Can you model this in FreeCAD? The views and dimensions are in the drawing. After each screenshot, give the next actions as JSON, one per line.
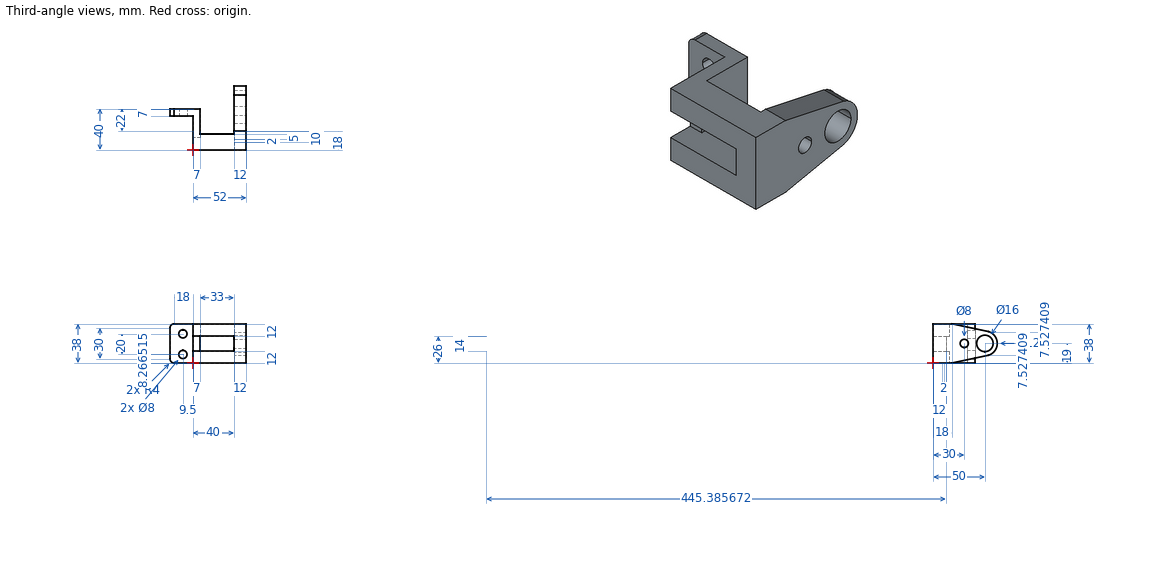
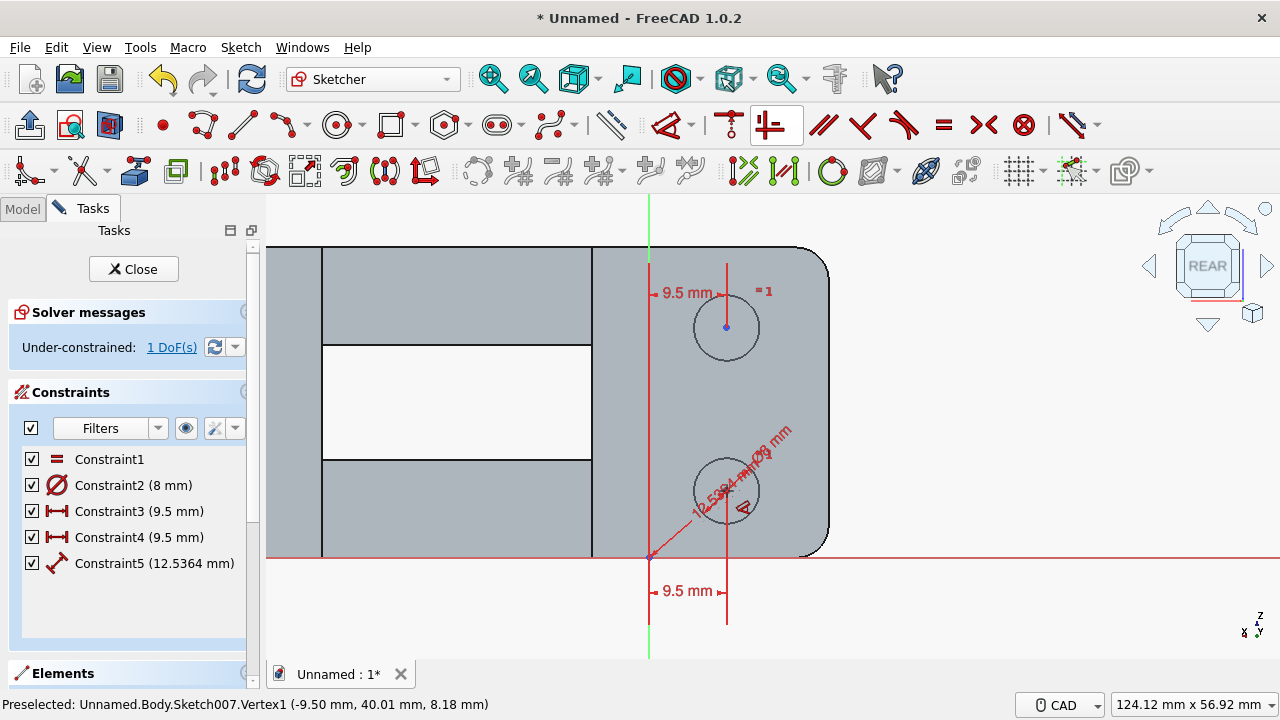
{"action": "left_click", "coordinate": [727, 328]}
{"action": "left_click", "coordinate": [761, 410]}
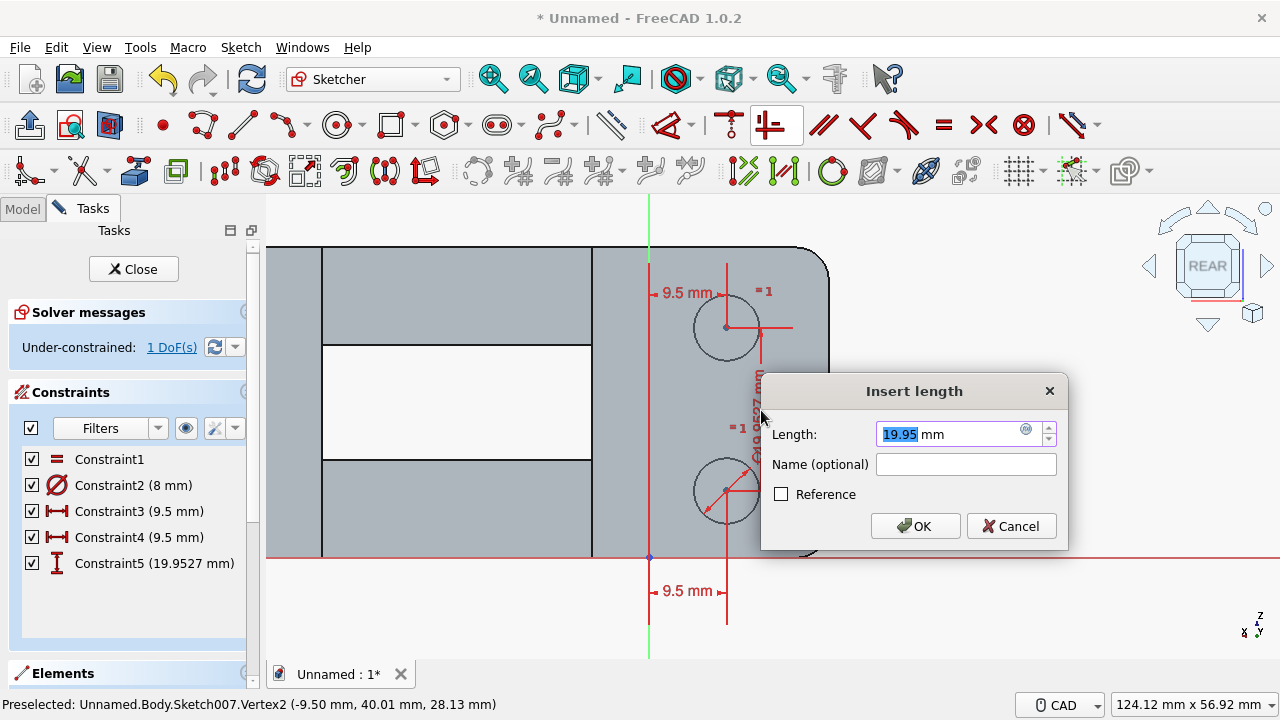
{"action": "type", "text": "20"}
{"action": "key", "text": "Return"}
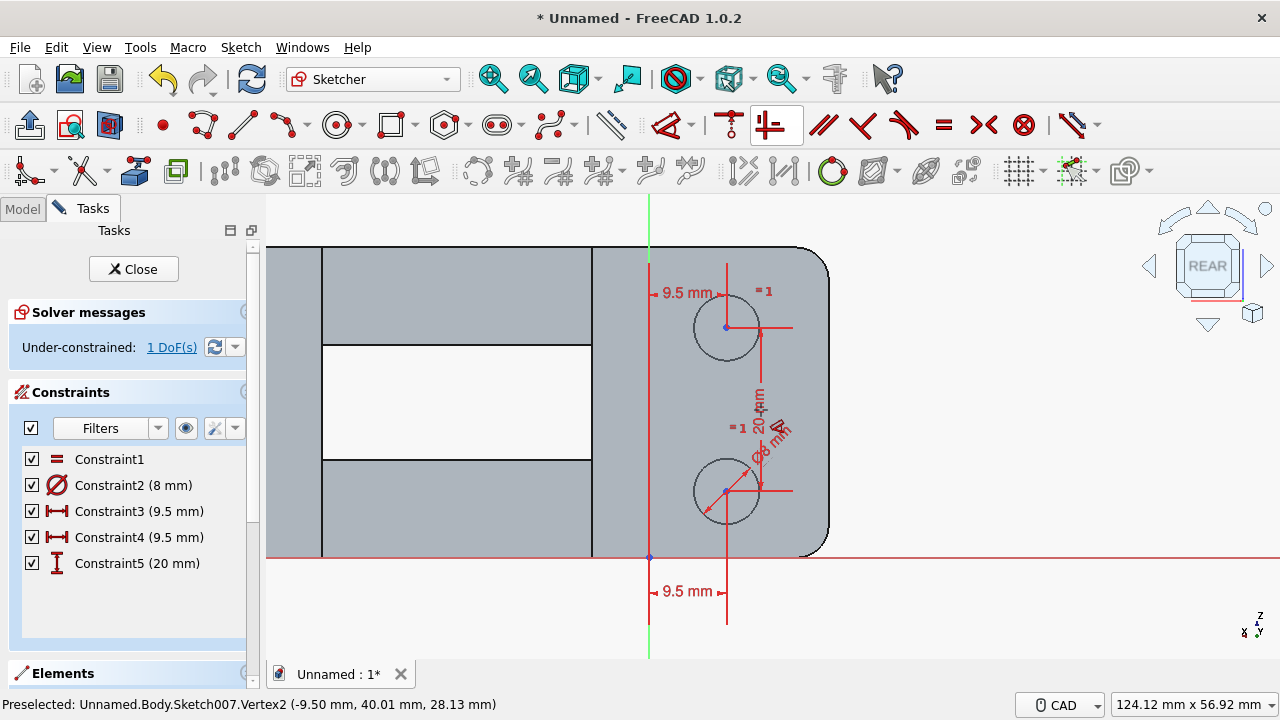
{"action": "left_click", "coordinate": [727, 491]}
{"action": "left_click", "coordinate": [615, 525]}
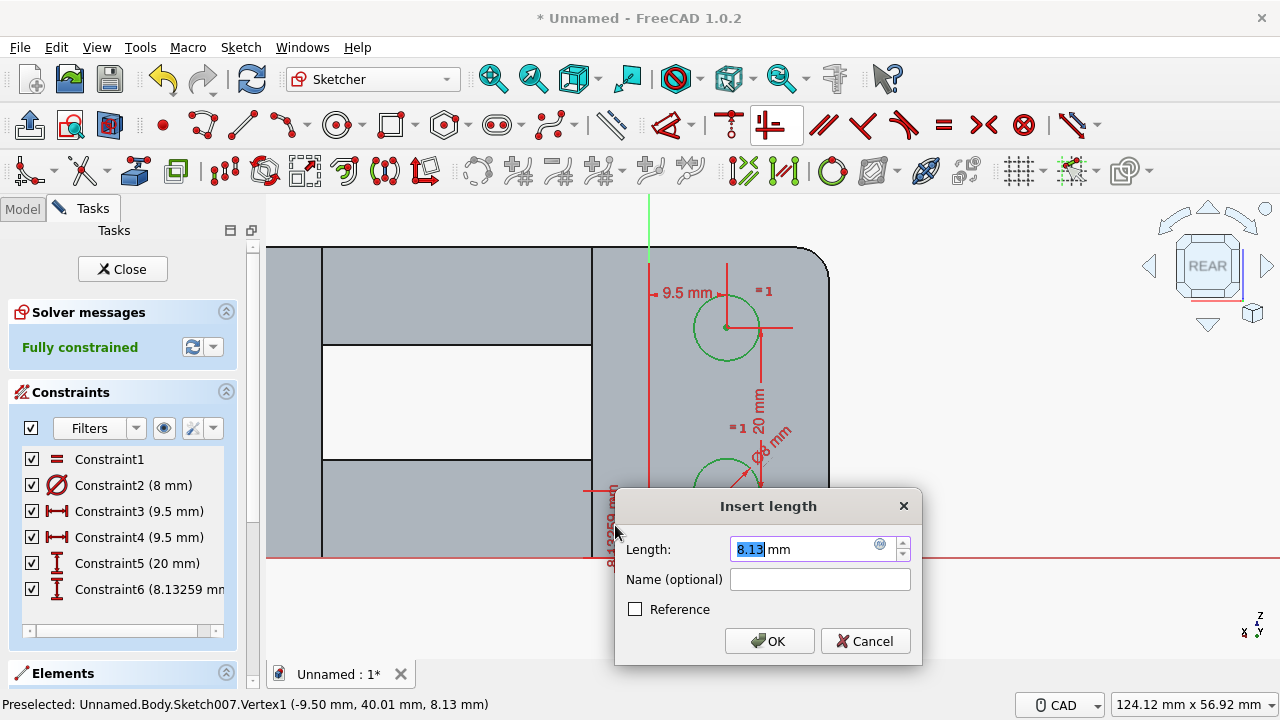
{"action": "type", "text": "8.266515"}
{"action": "key", "text": "Return"}
{"action": "key", "text": "Escape"}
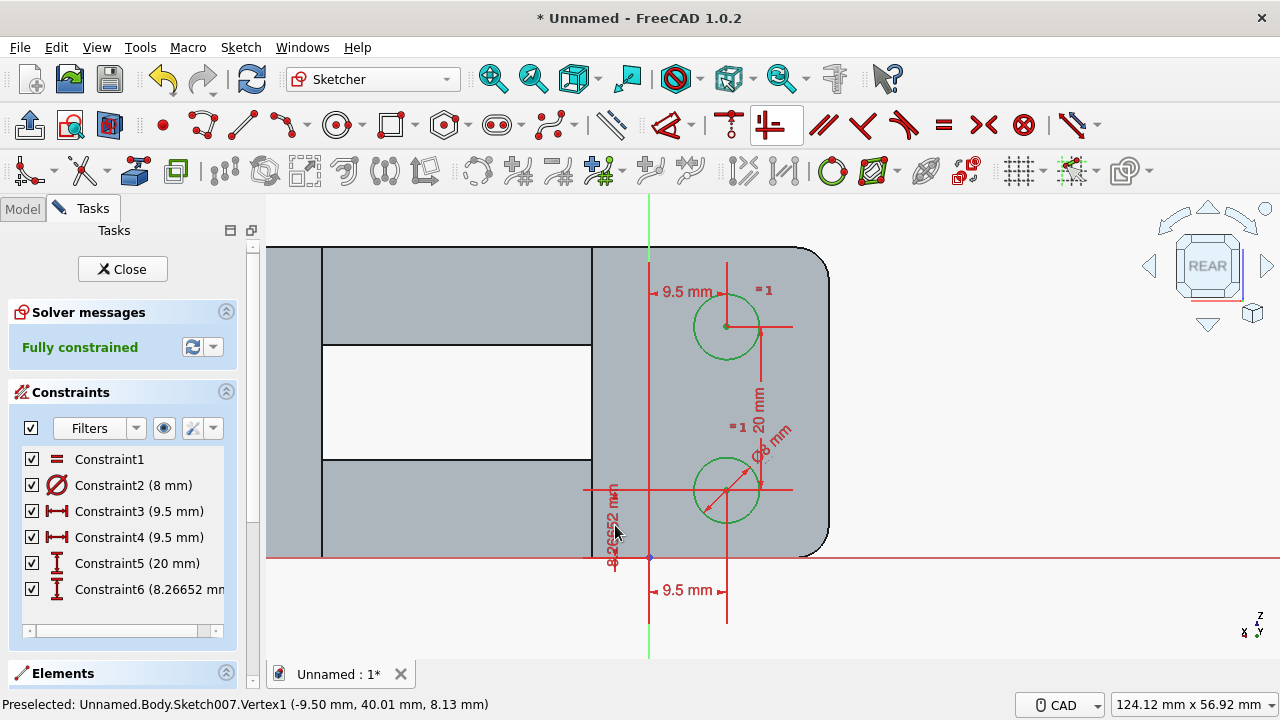
{"action": "left_click", "coordinate": [123, 269]}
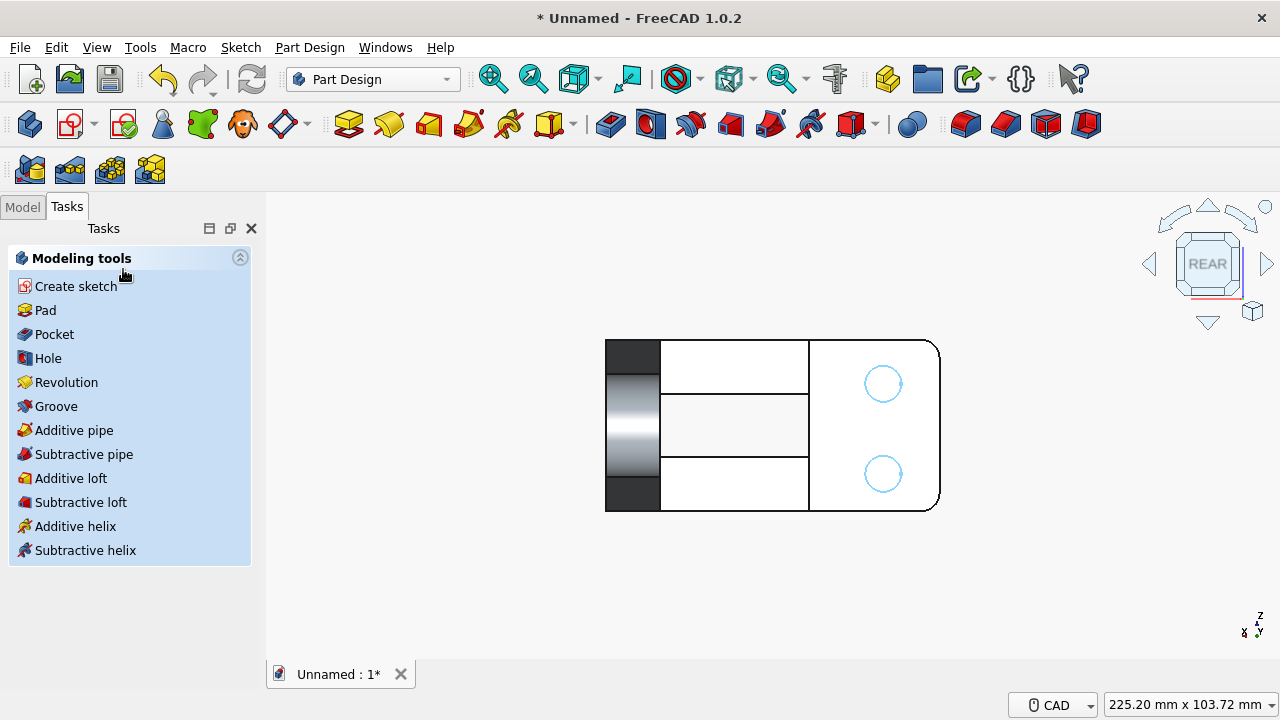
{"action": "left_click", "coordinate": [612, 124]}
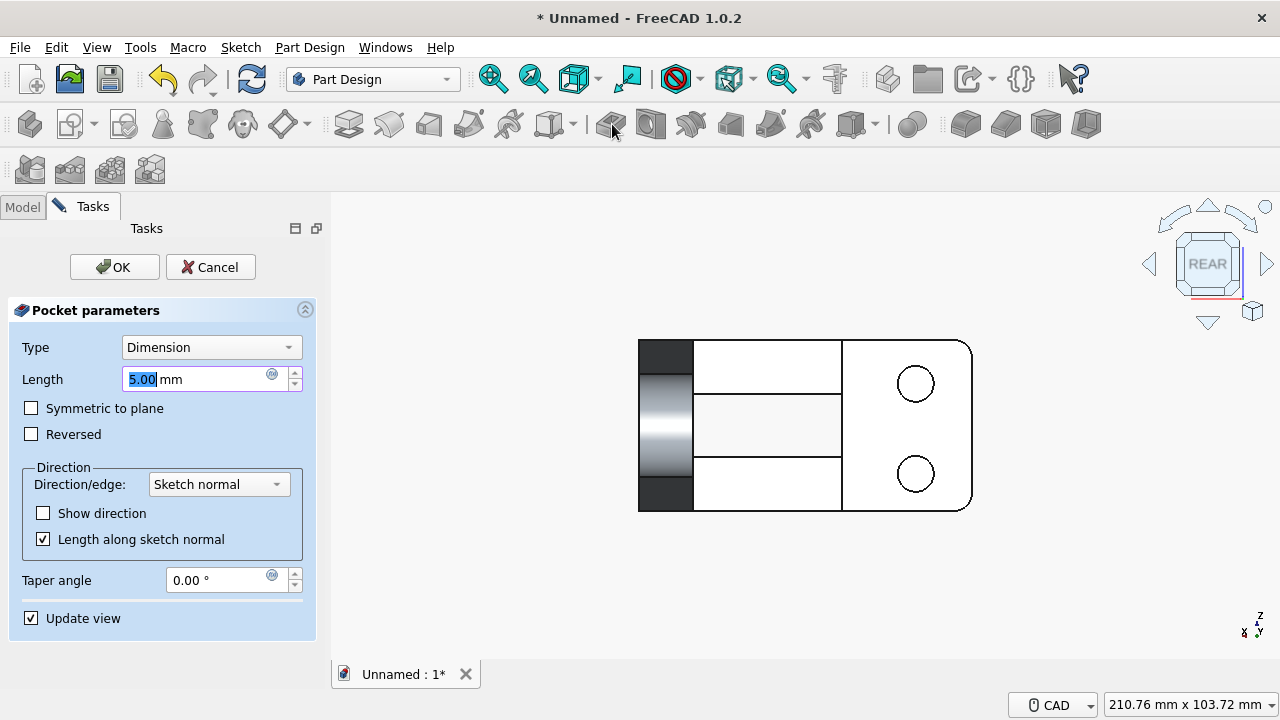
{"action": "type", "text": "7"}
{"action": "key", "text": "Tab"}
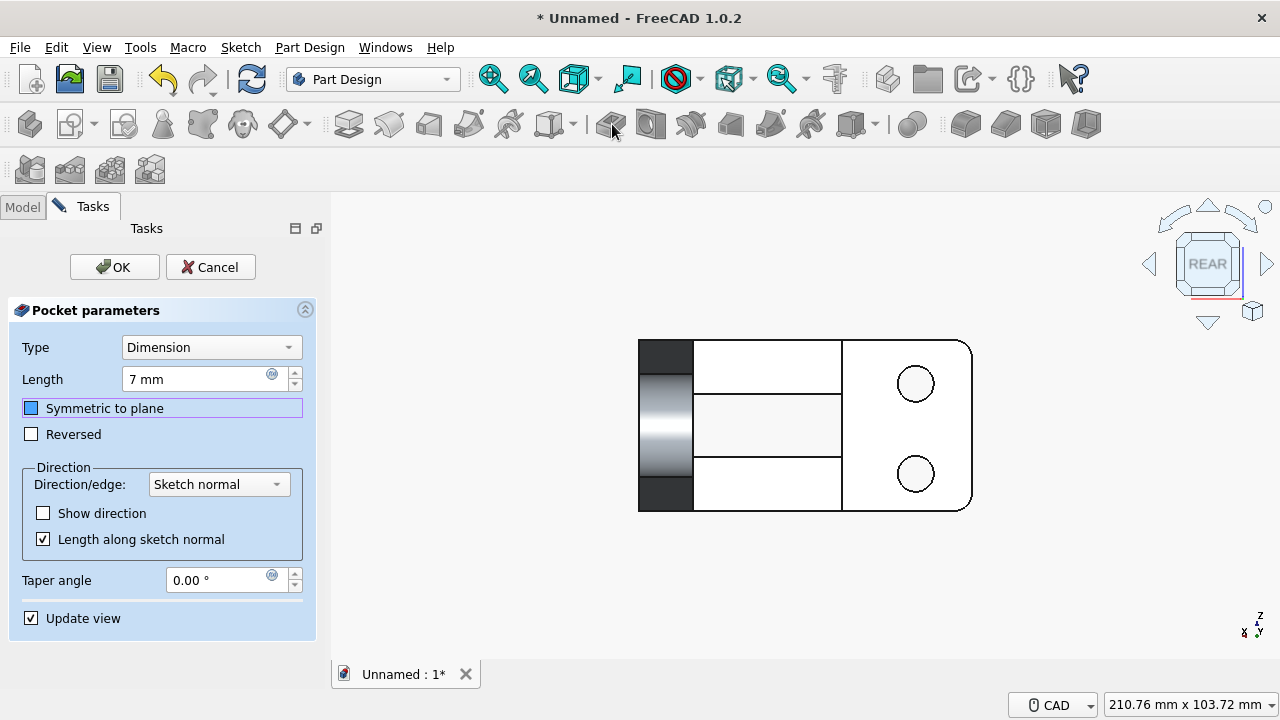
{"action": "left_click", "coordinate": [115, 267]}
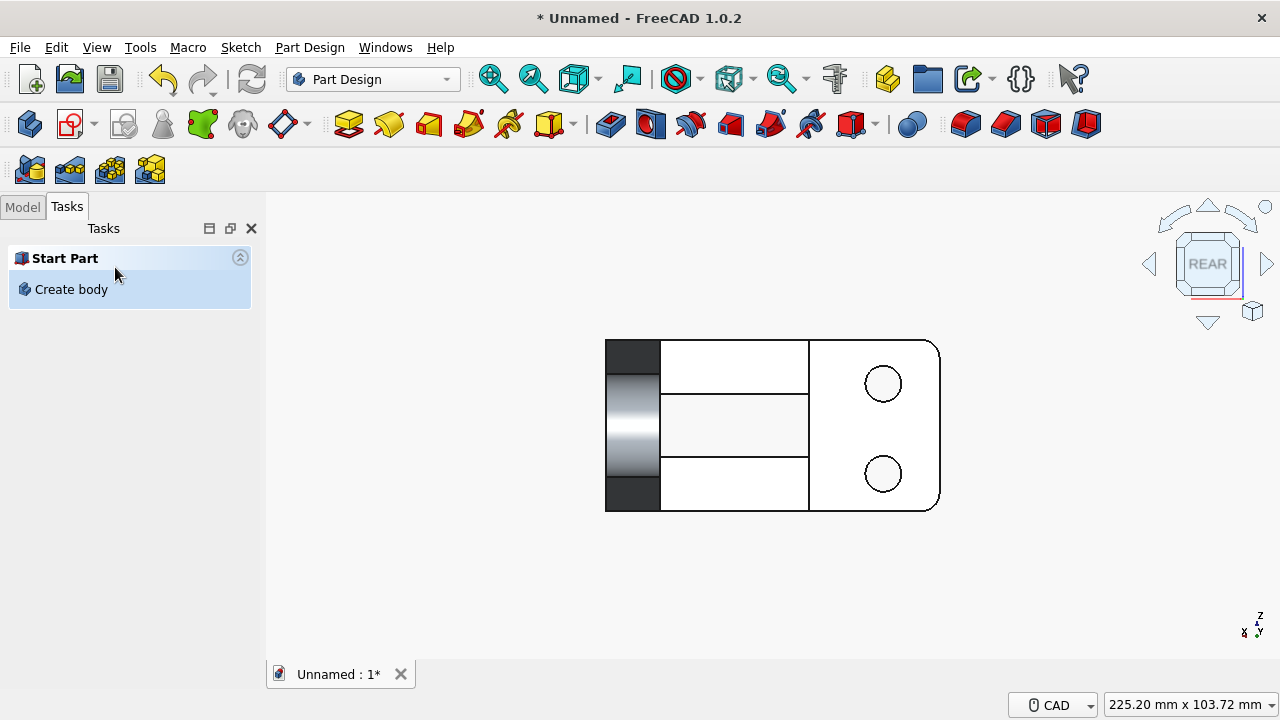
{"action": "left_click", "coordinate": [494, 80]}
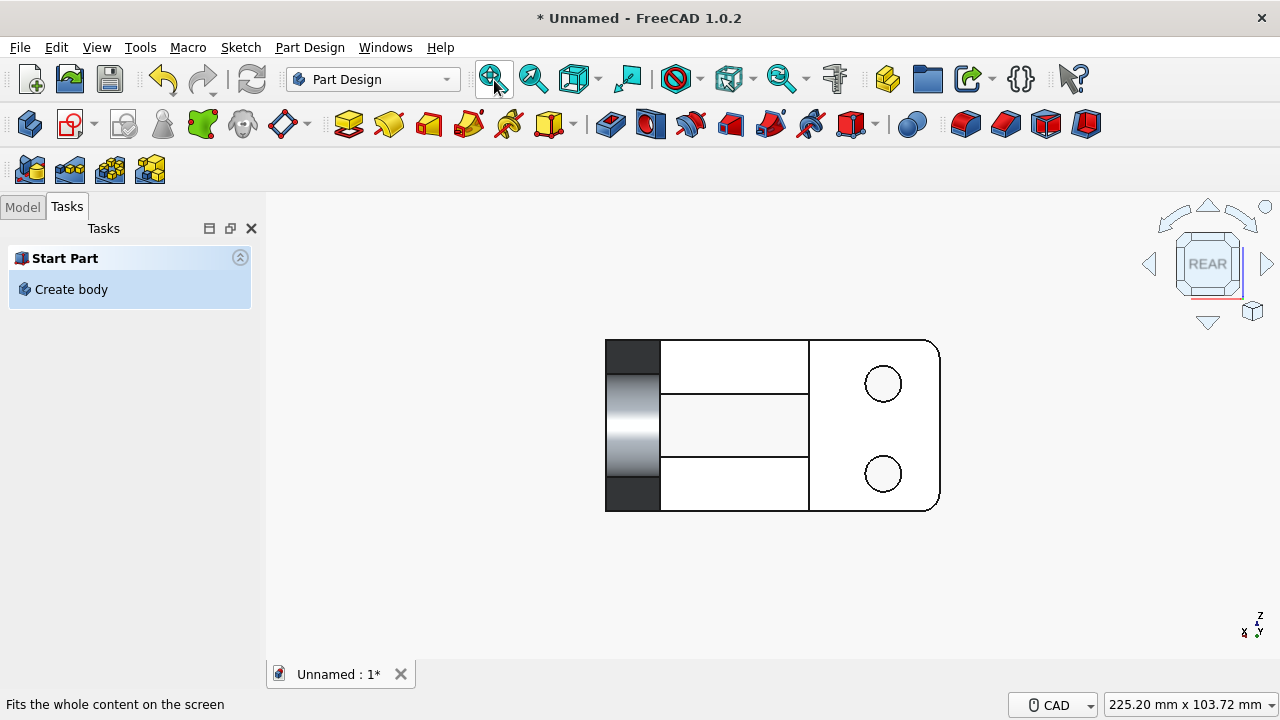
{"action": "key", "text": "0"}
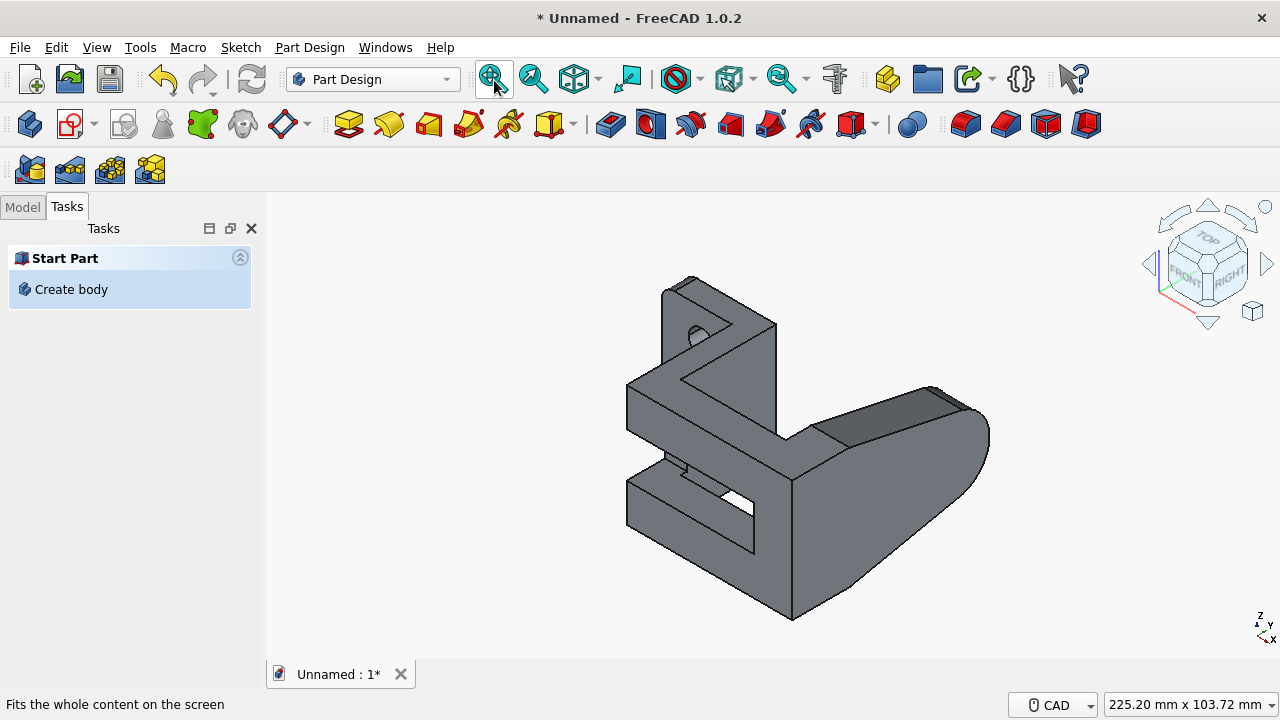
{"action": "left_click", "coordinate": [863, 509]}